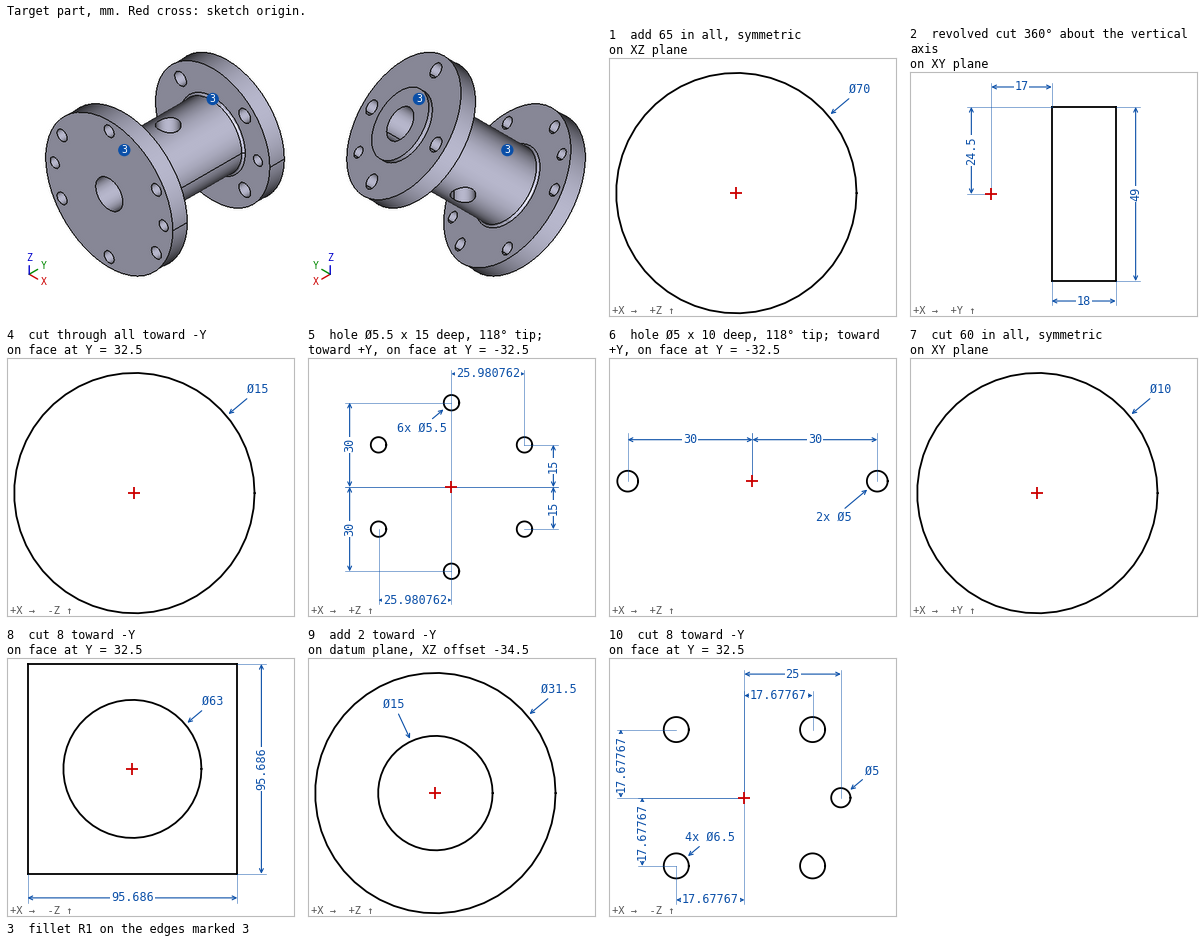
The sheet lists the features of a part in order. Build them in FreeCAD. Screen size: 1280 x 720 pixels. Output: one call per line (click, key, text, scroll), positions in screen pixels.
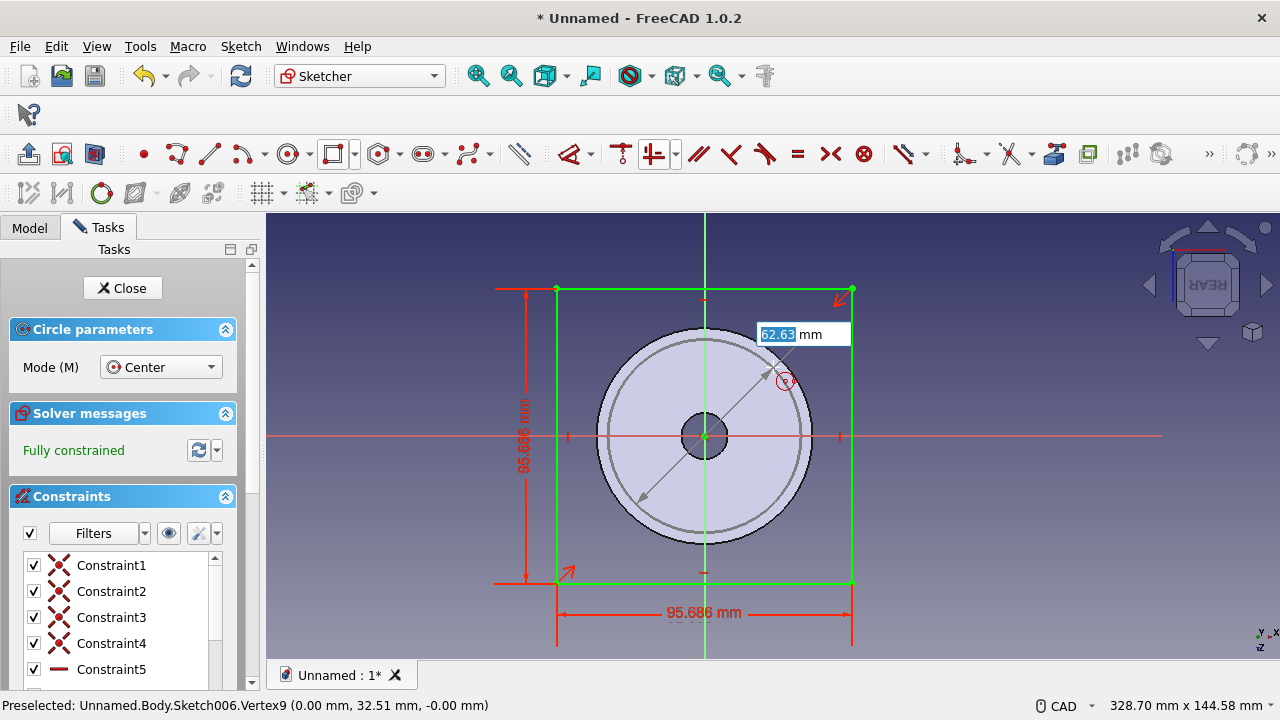
text(63)
key(Return)
key(Escape)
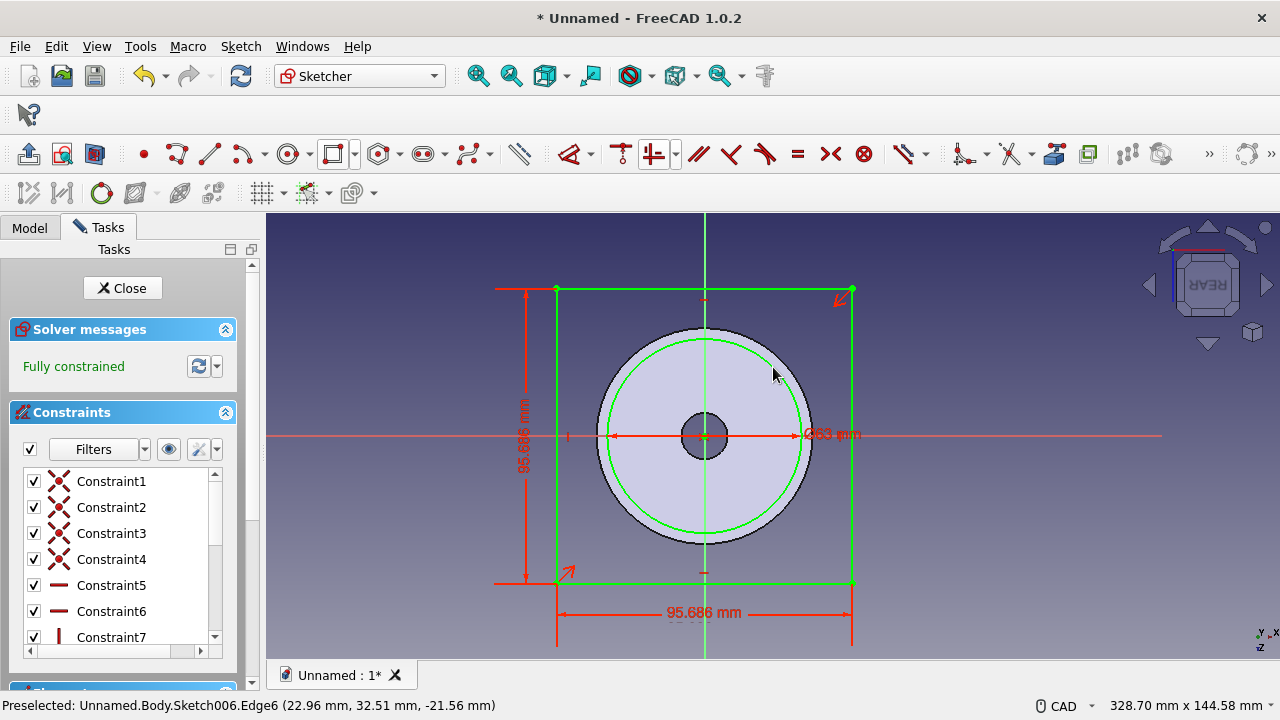
click(123, 288)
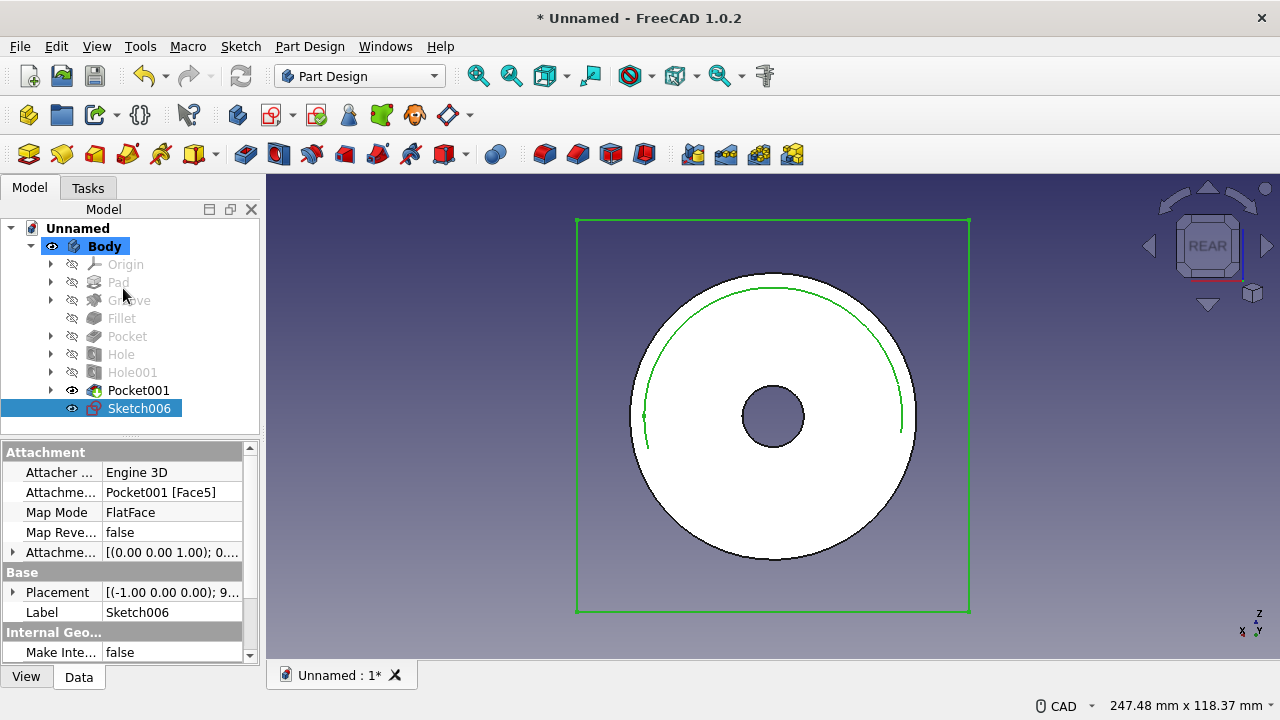
click(246, 154)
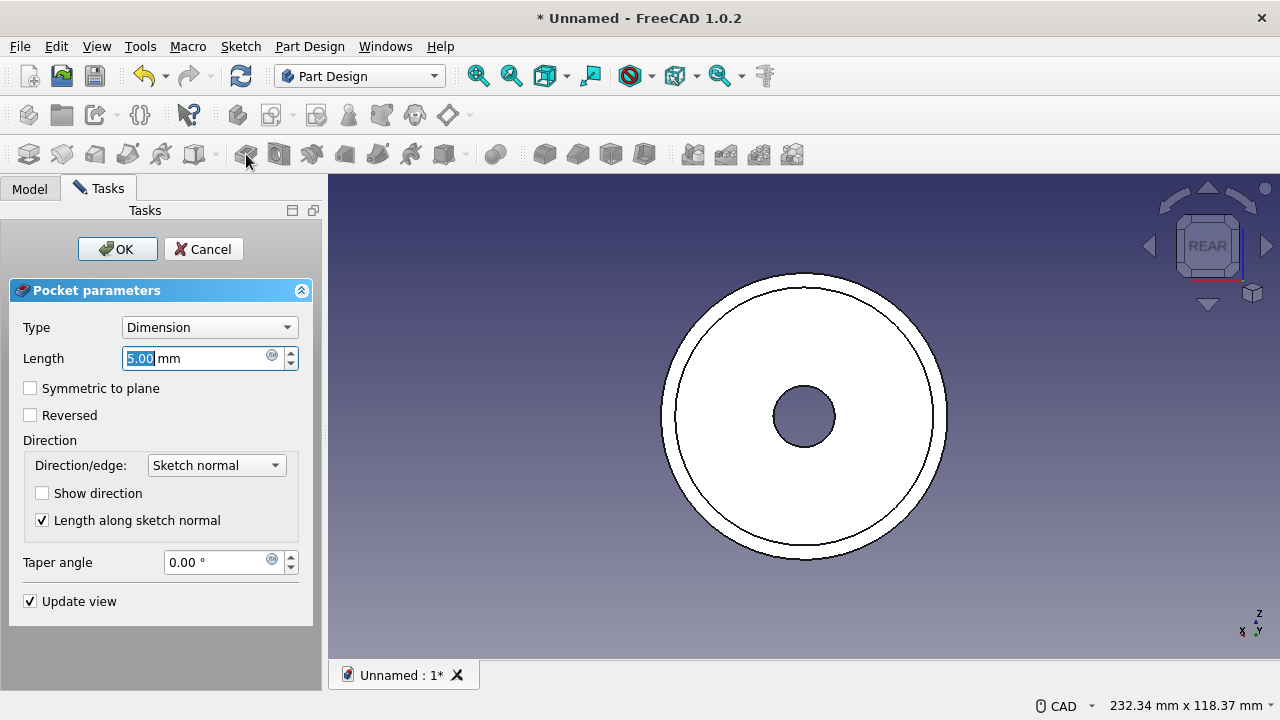
text(8)
key(Tab)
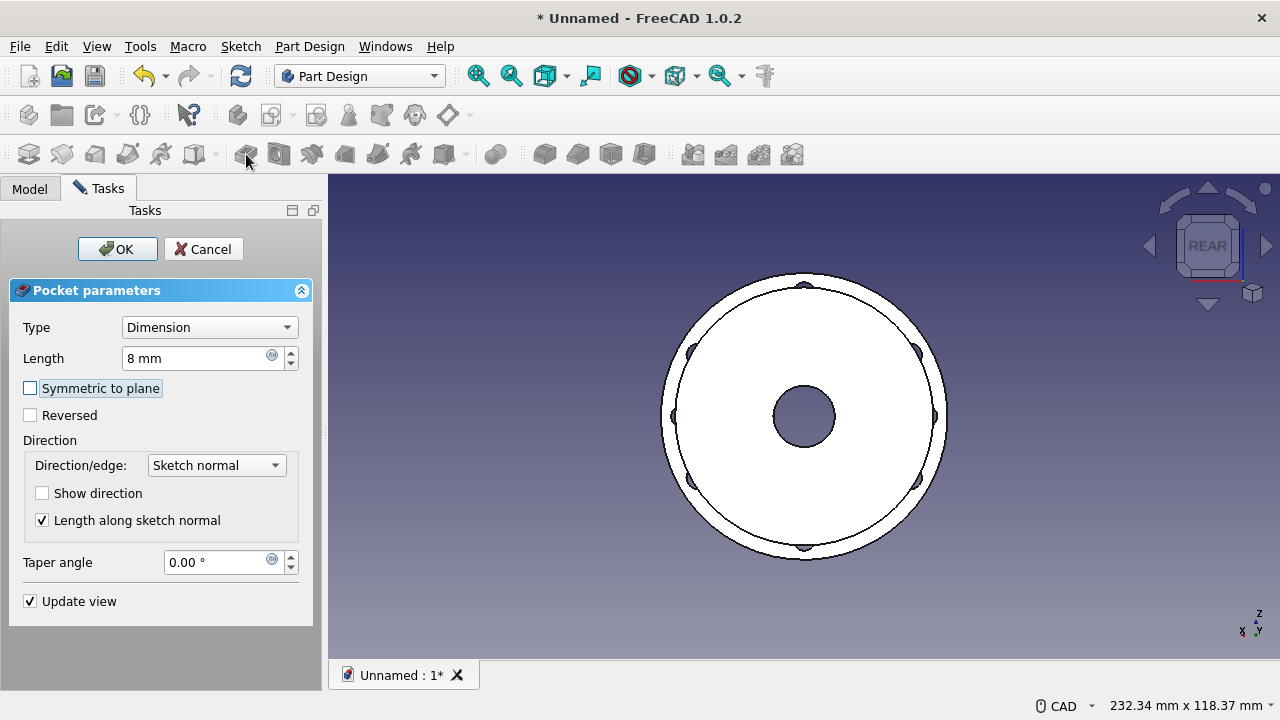
click(118, 249)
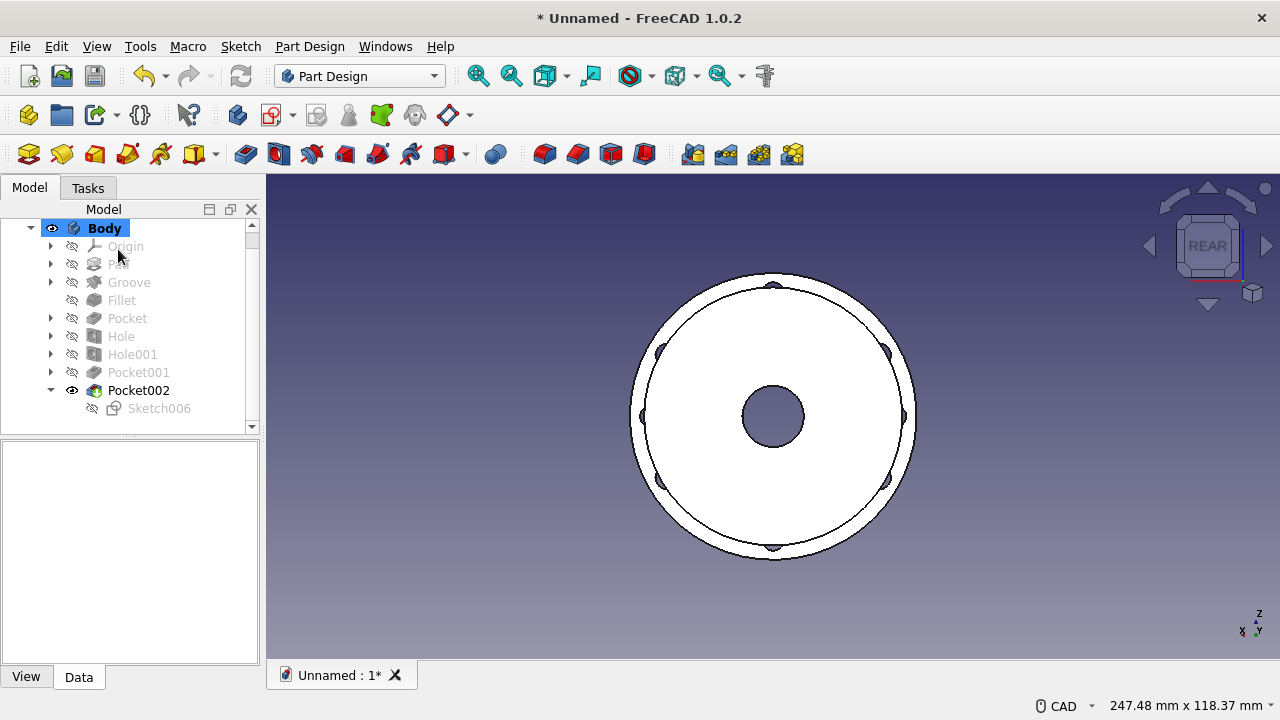
click(51, 246)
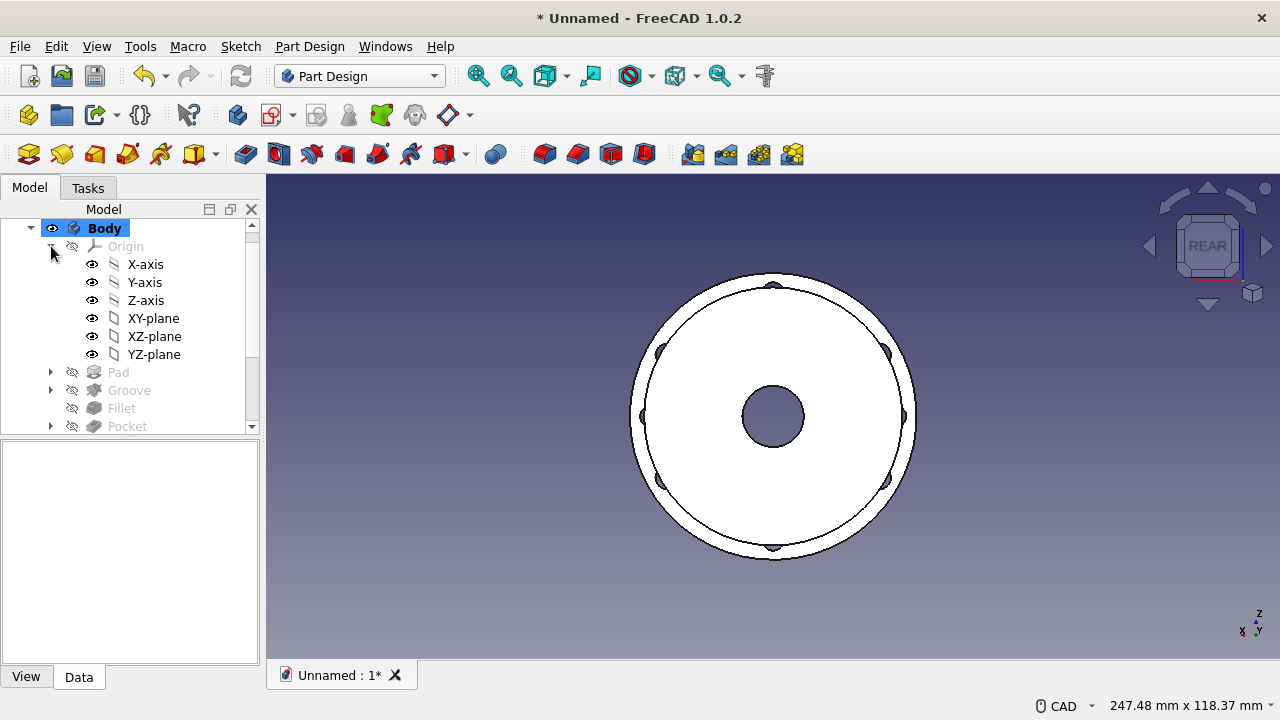
click(137, 336)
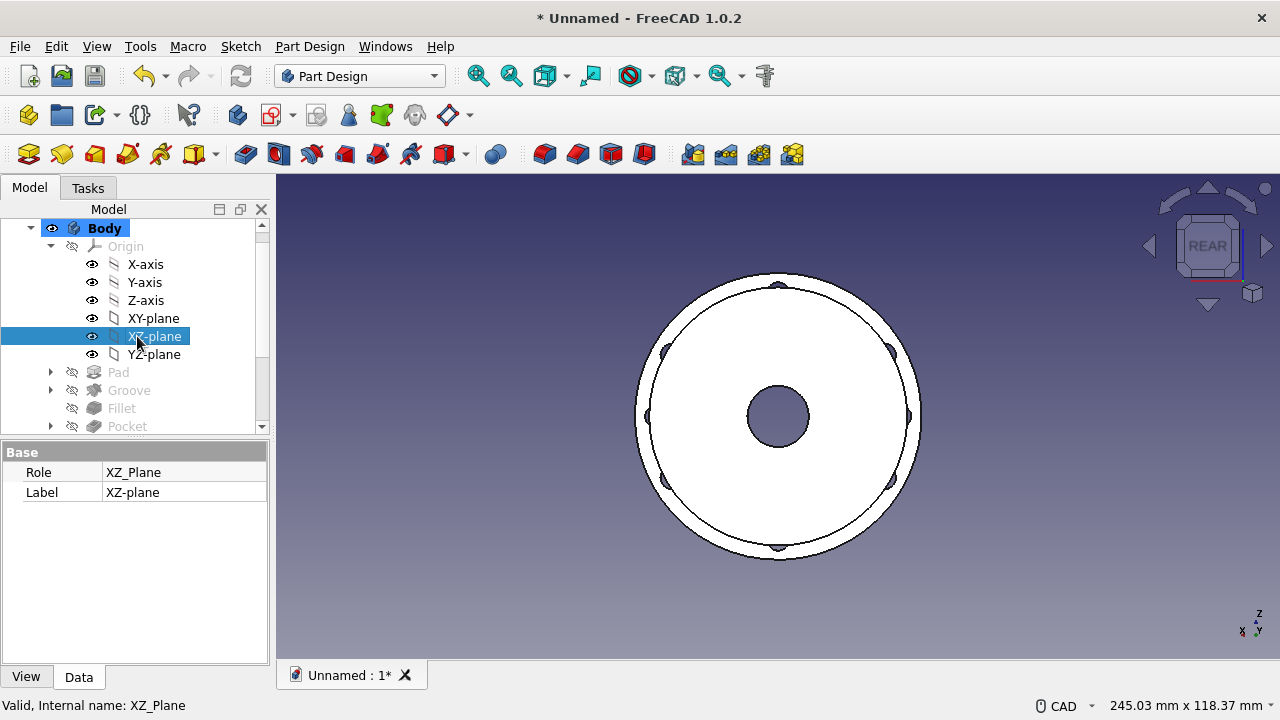
click(448, 116)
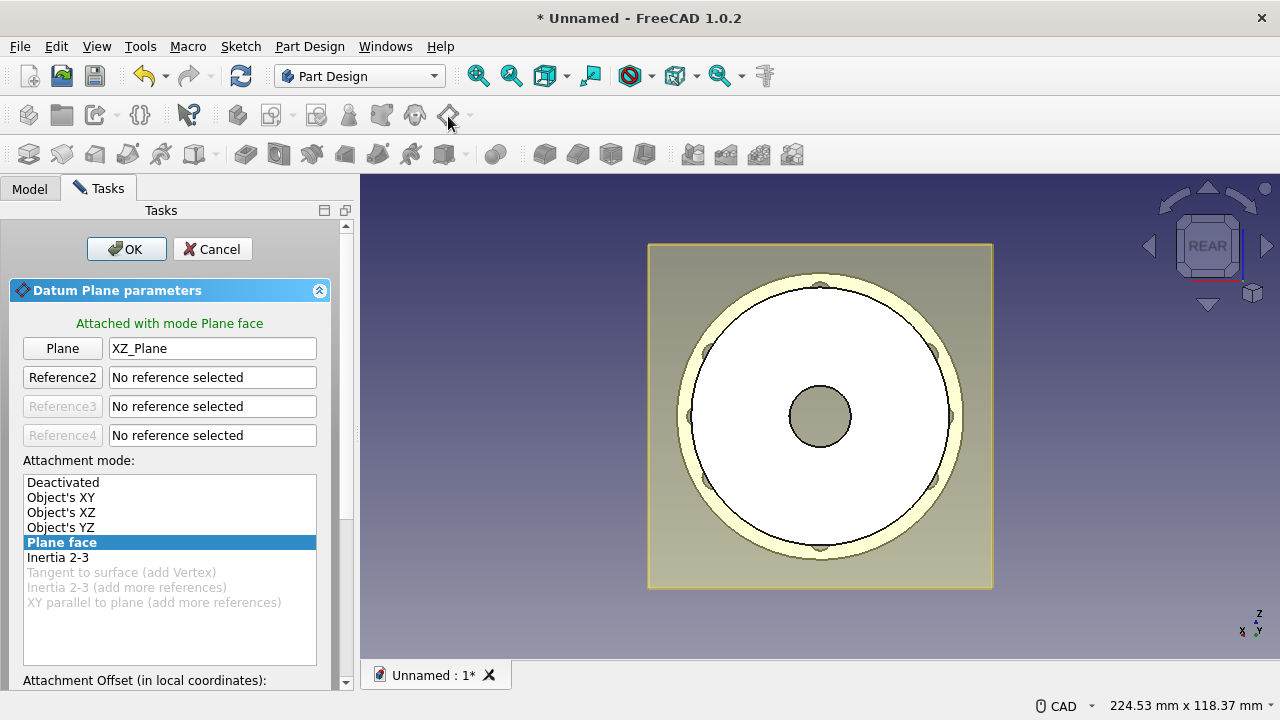
scroll(346, 455, down, 3)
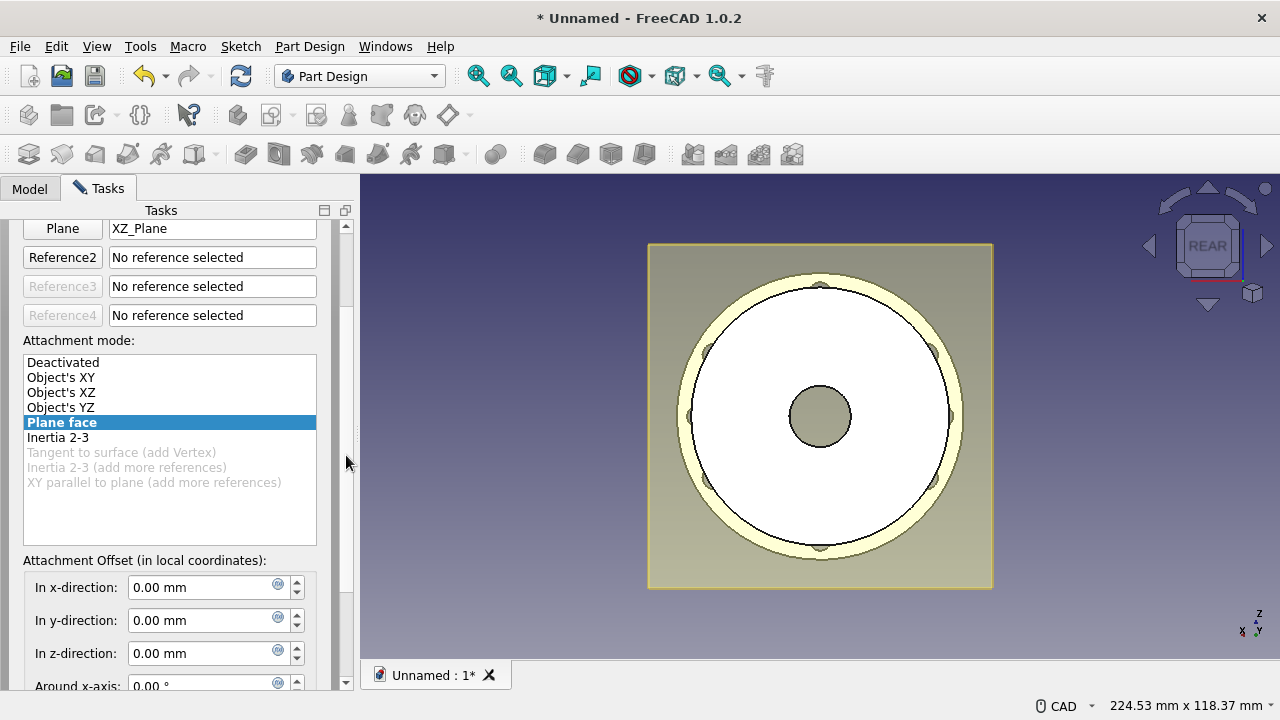
triple_click(210, 594)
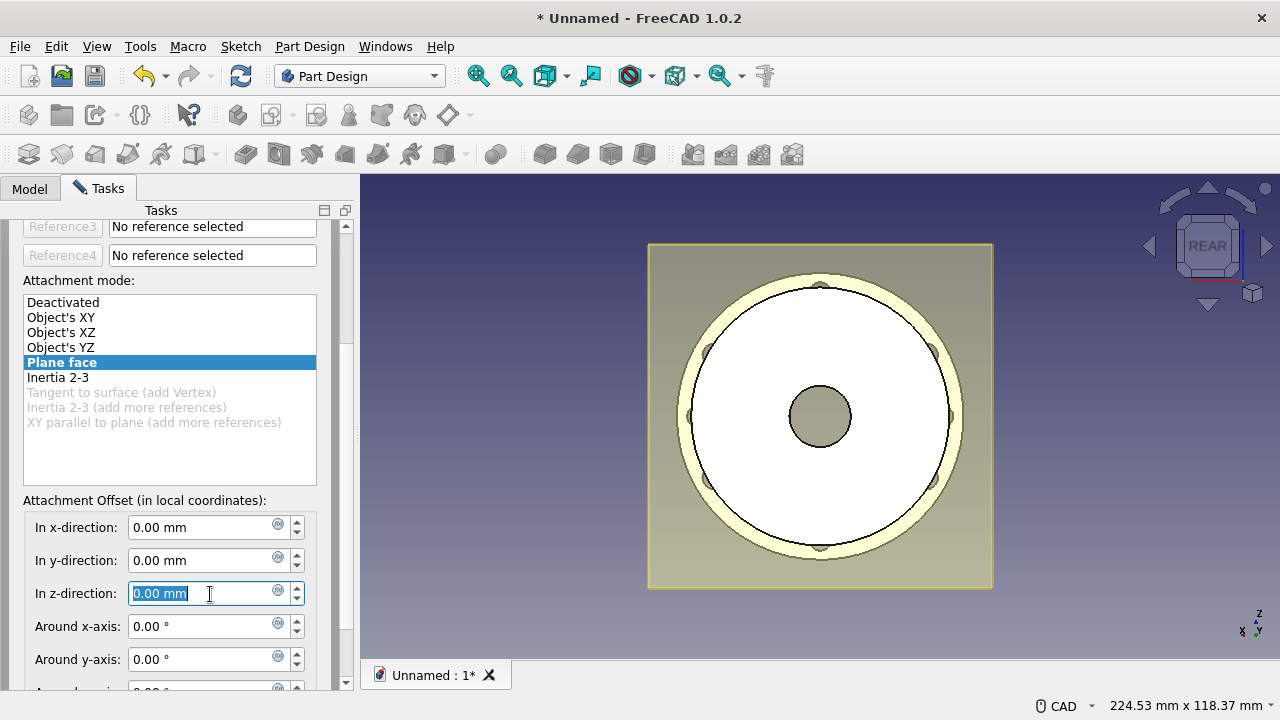
text(-34.5)
key(Tab)